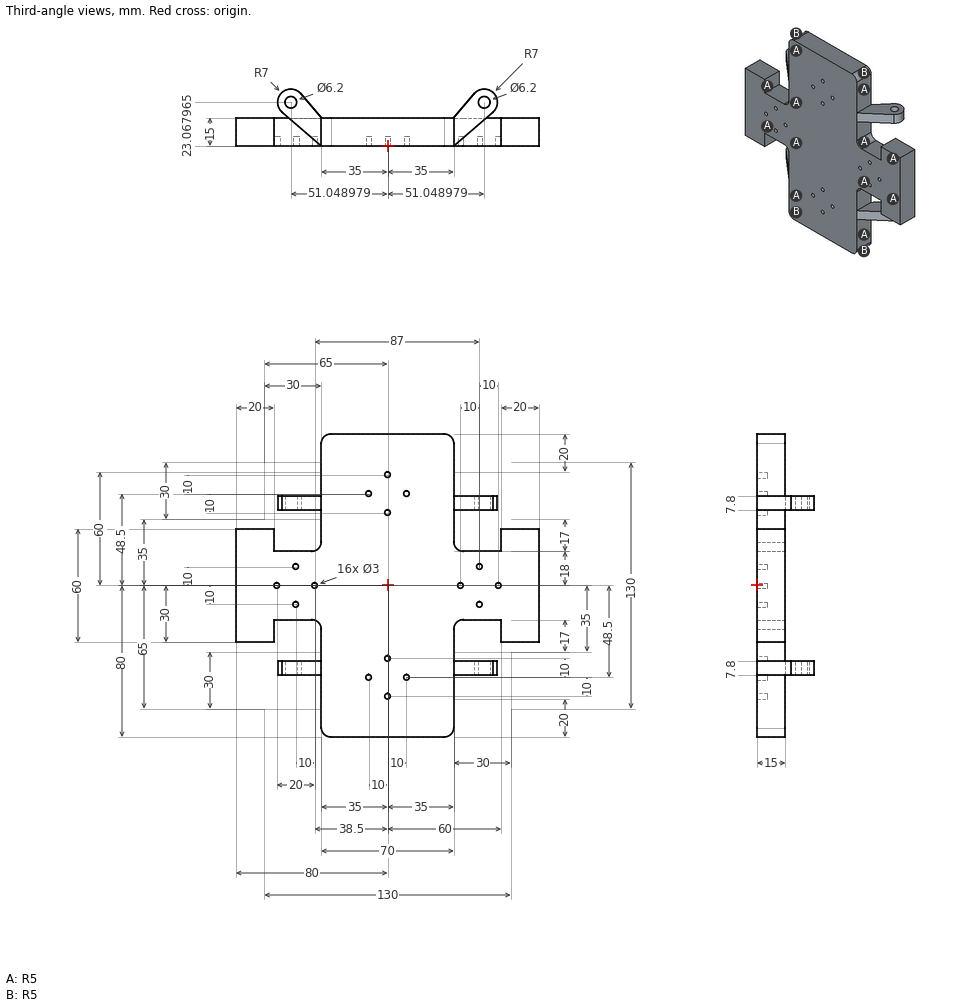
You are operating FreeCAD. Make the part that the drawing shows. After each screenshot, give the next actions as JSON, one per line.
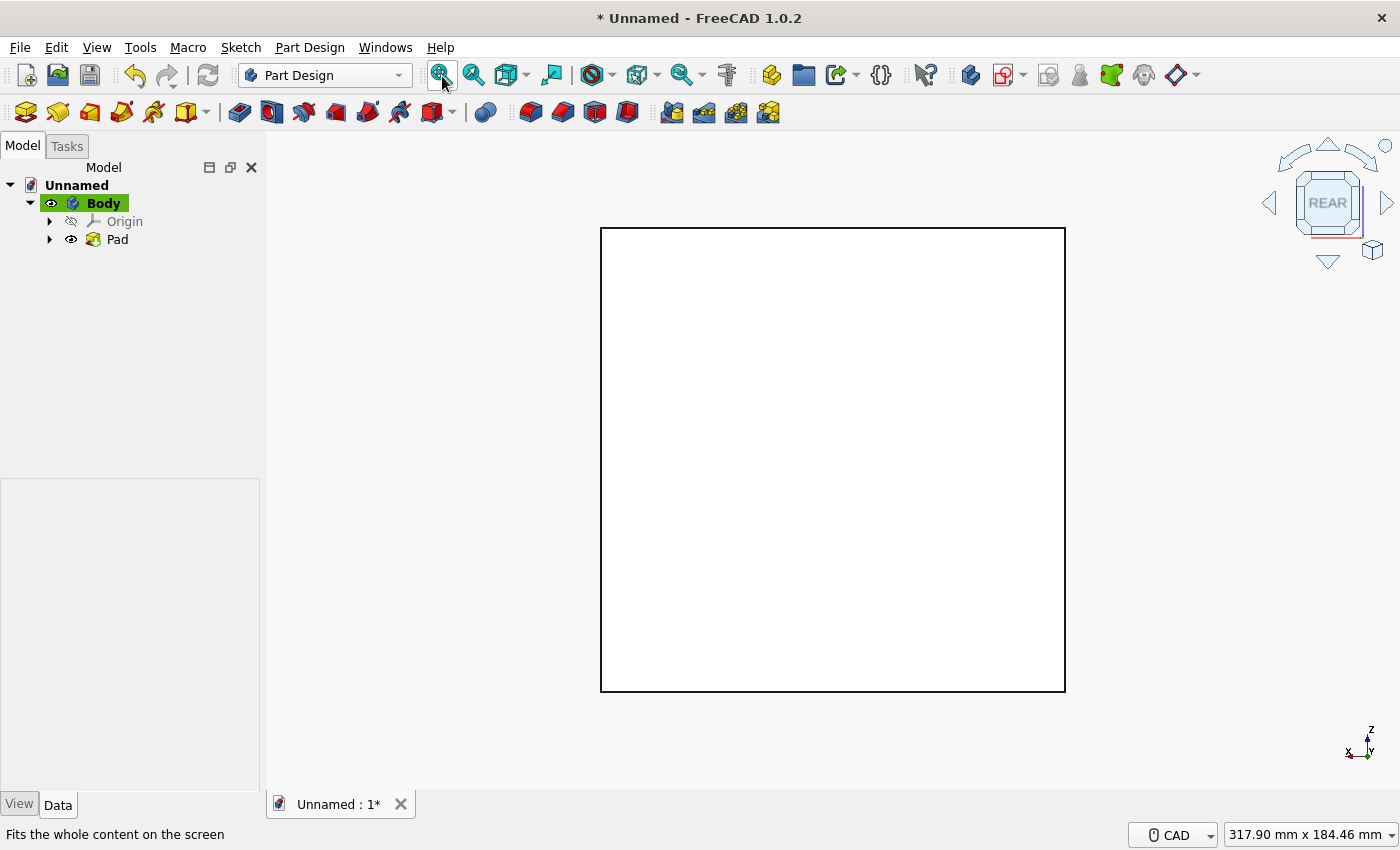
{"action": "left_click", "coordinate": [833, 459]}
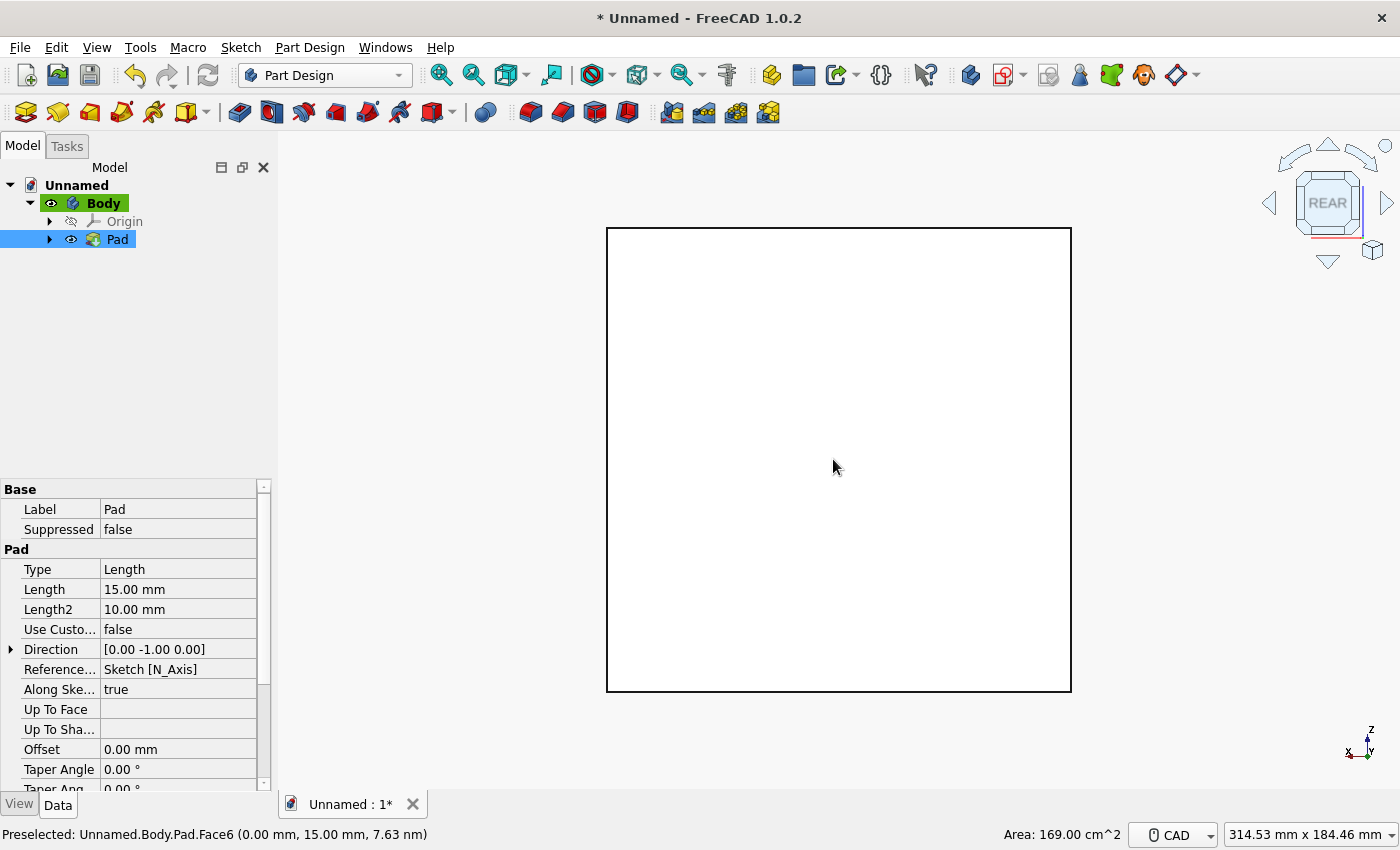
{"action": "left_click", "coordinate": [1004, 76]}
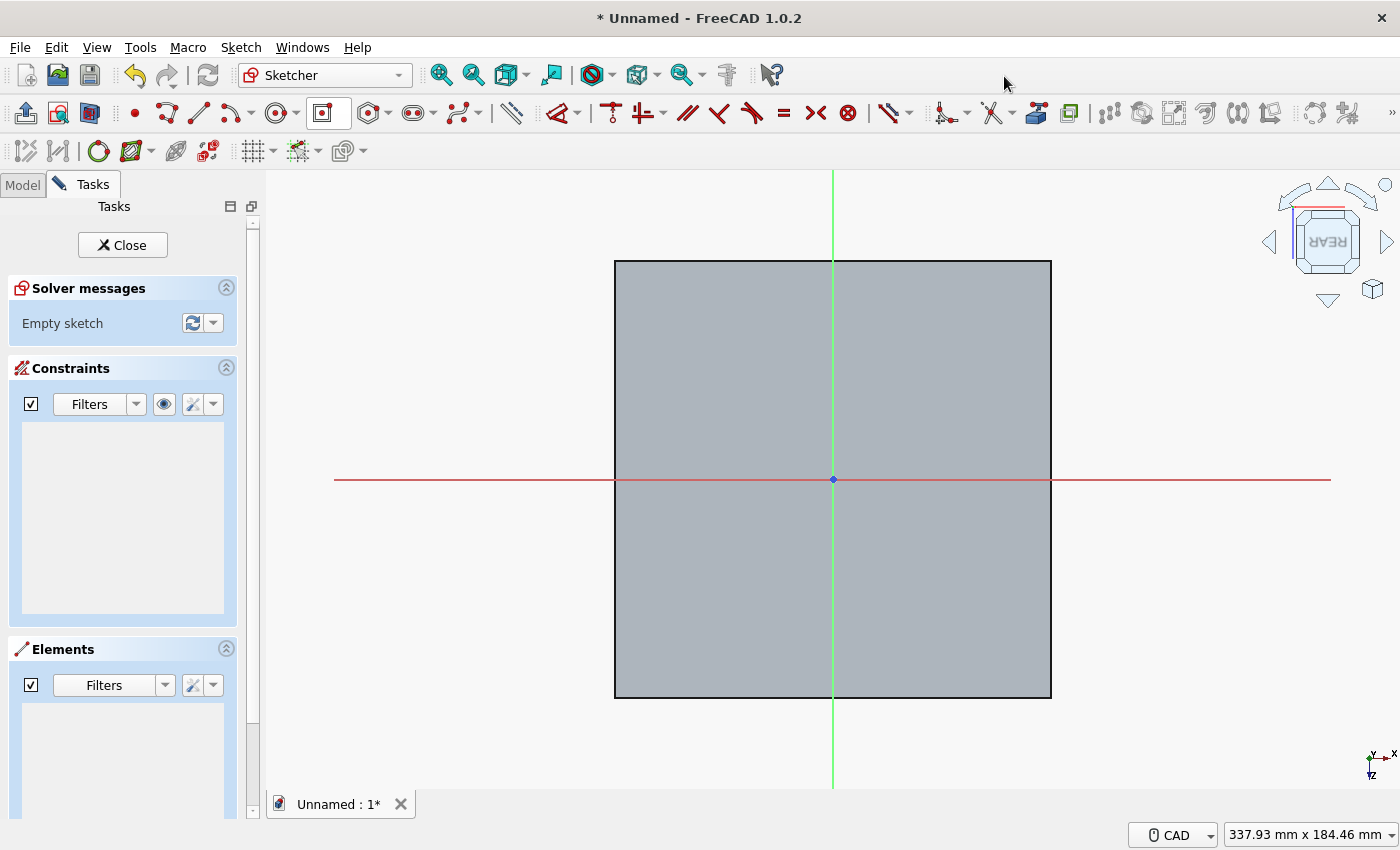
{"action": "key", "text": "g r"}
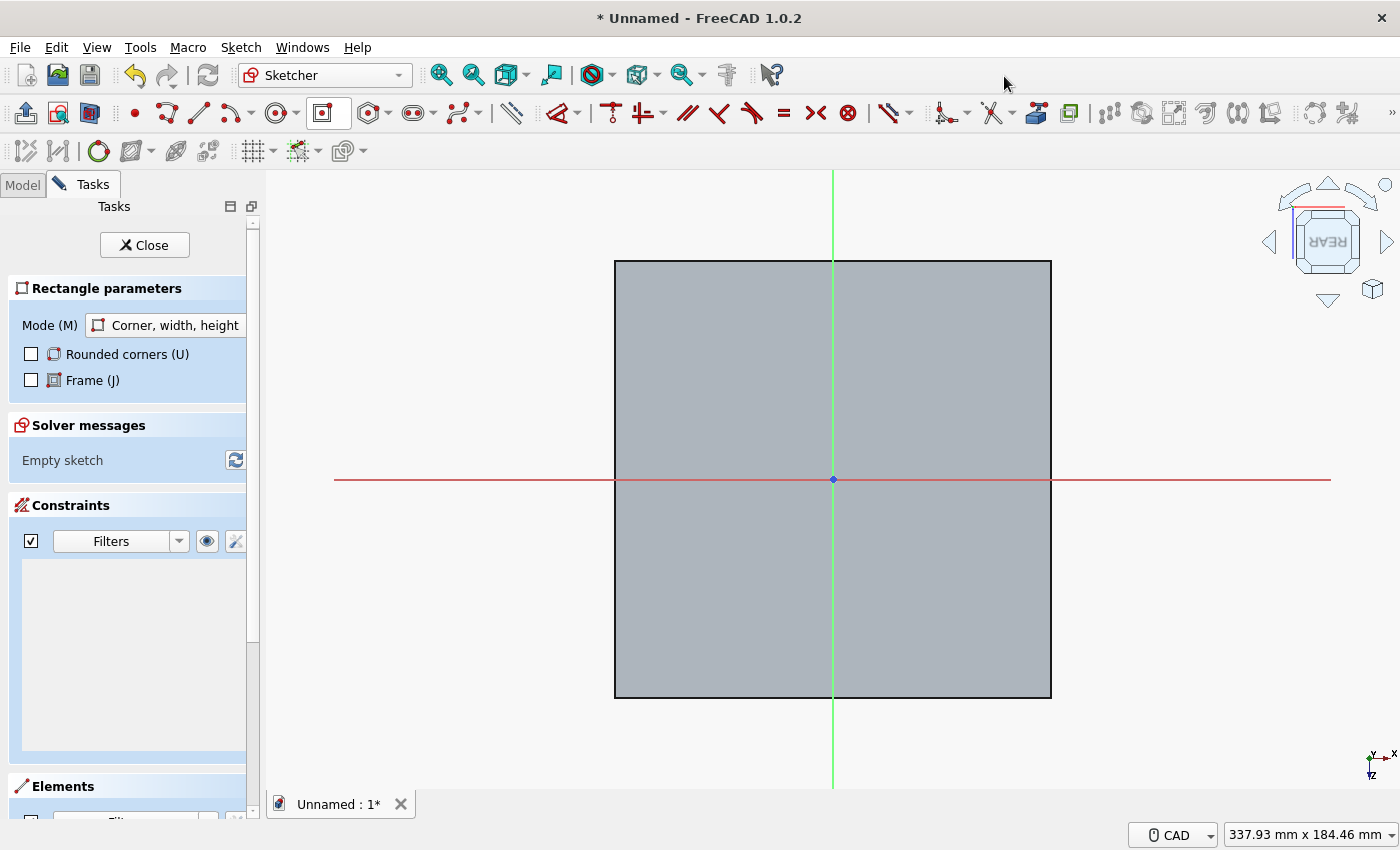
{"action": "left_click", "coordinate": [615, 597]}
{"action": "mouse_move", "coordinate": [716, 698]}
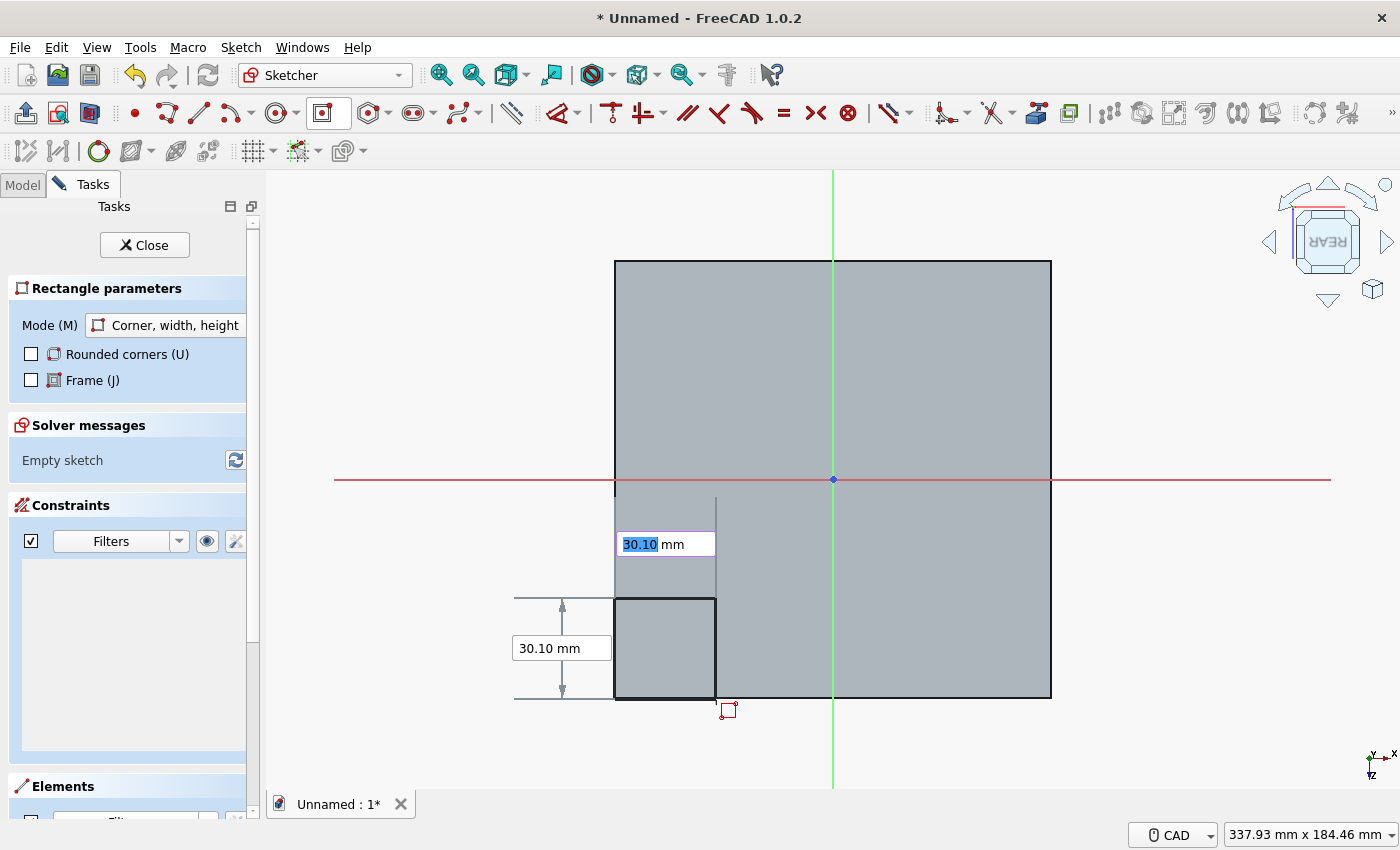
{"action": "type", "text": "30"}
{"action": "key", "text": "Tab"}
{"action": "type", "text": "30"}
{"action": "key", "text": "Return"}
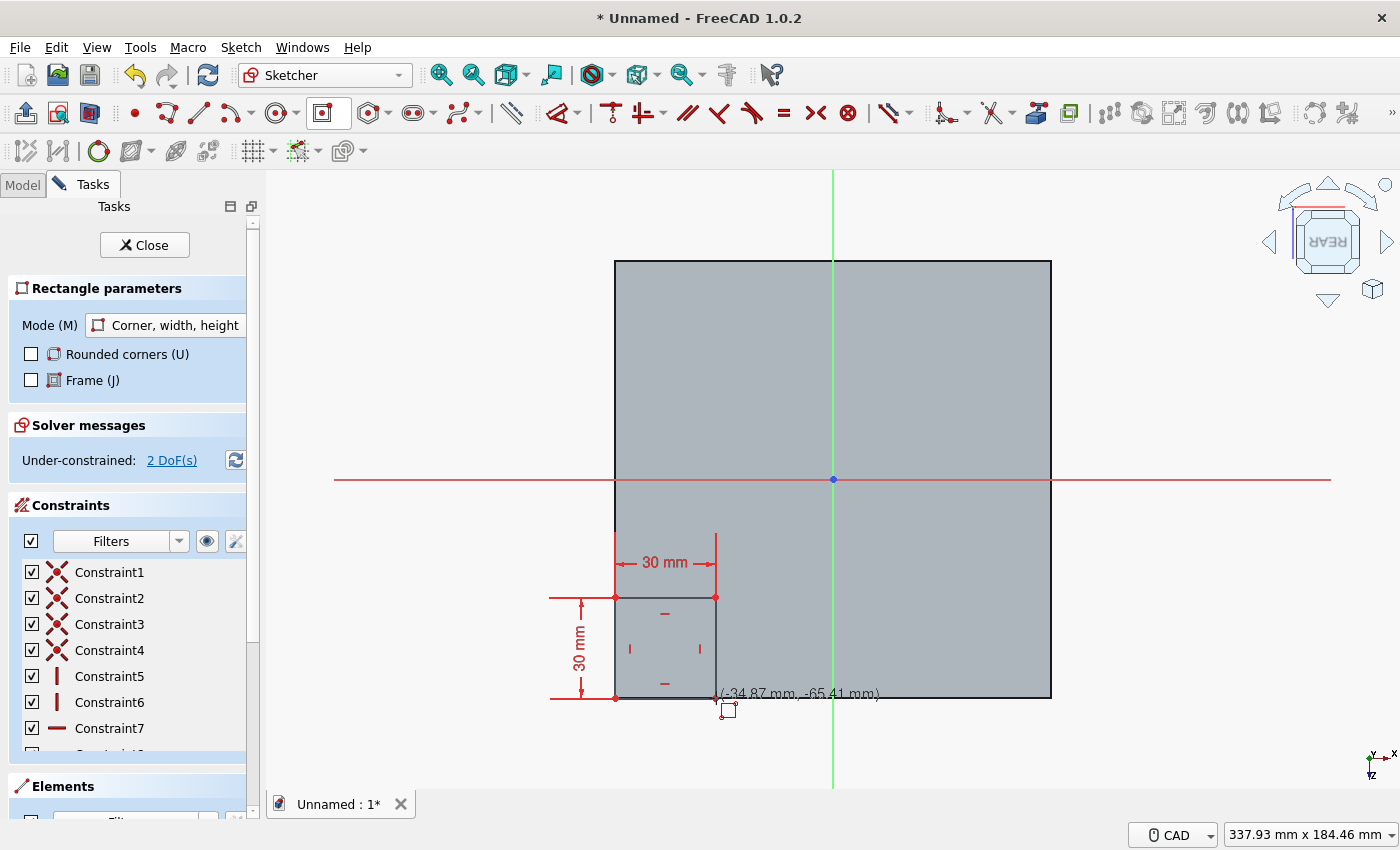
{"action": "left_click", "coordinate": [615, 261]}
{"action": "mouse_move", "coordinate": [716, 362]}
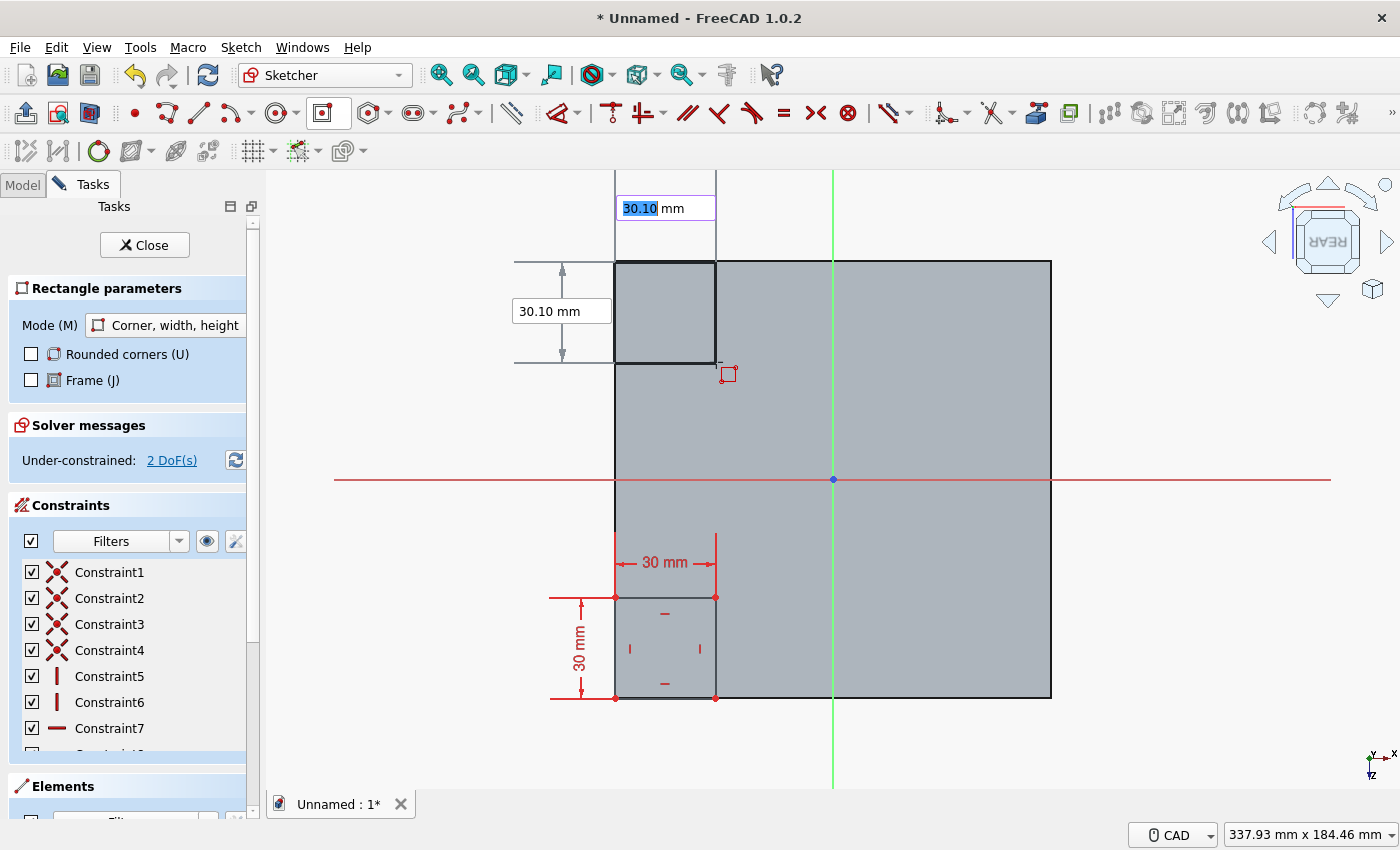
{"action": "type", "text": "30"}
{"action": "key", "text": "Tab"}
{"action": "type", "text": "30"}
{"action": "key", "text": "Return"}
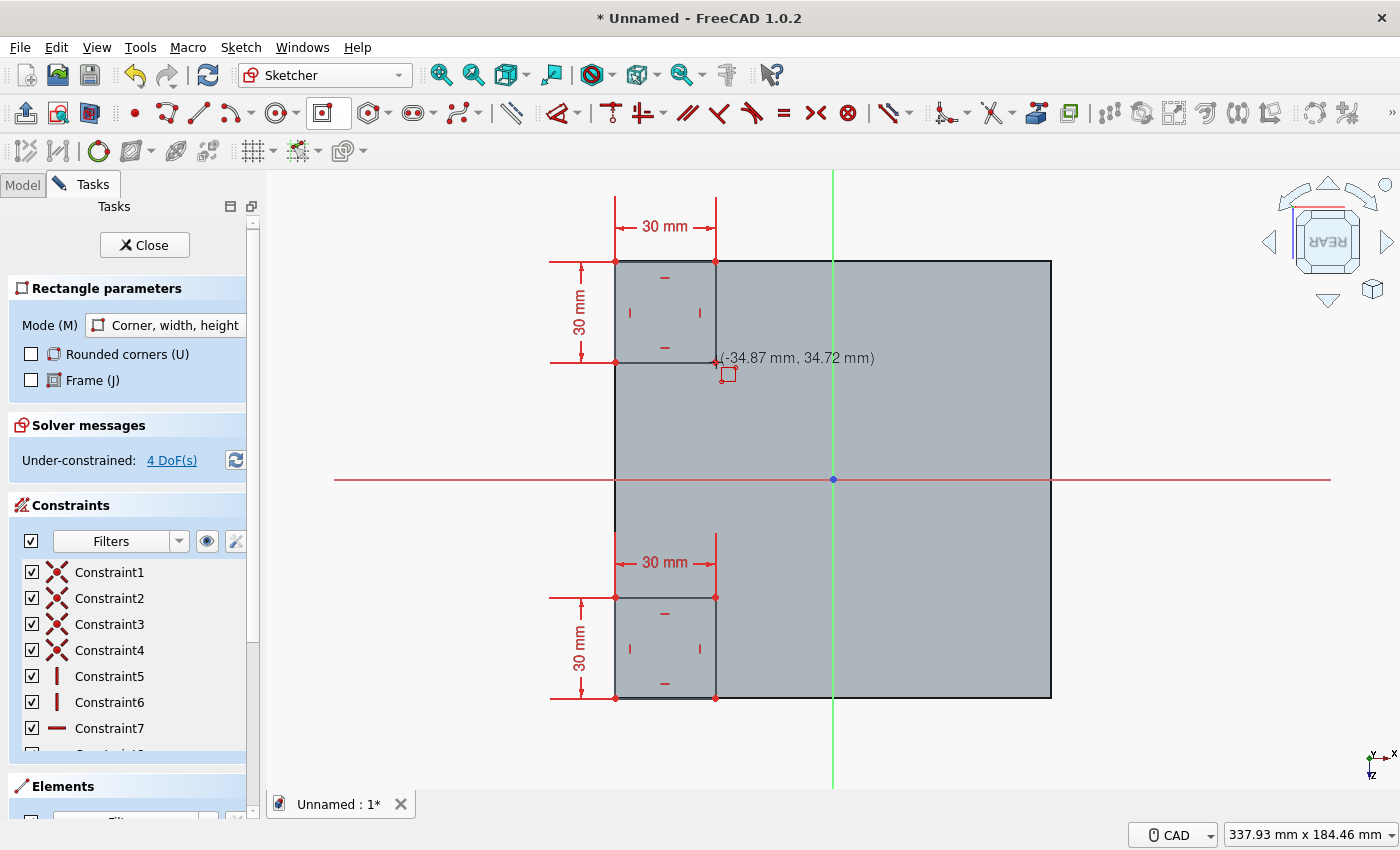
{"action": "left_click", "coordinate": [950, 261]}
{"action": "mouse_move", "coordinate": [1051, 362]}